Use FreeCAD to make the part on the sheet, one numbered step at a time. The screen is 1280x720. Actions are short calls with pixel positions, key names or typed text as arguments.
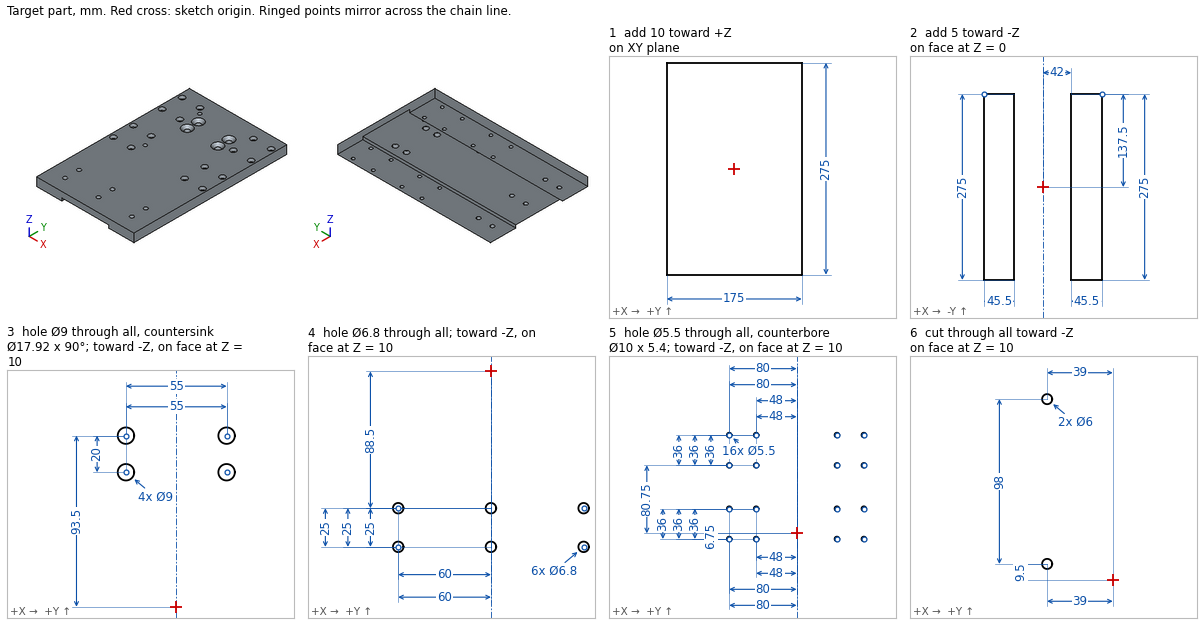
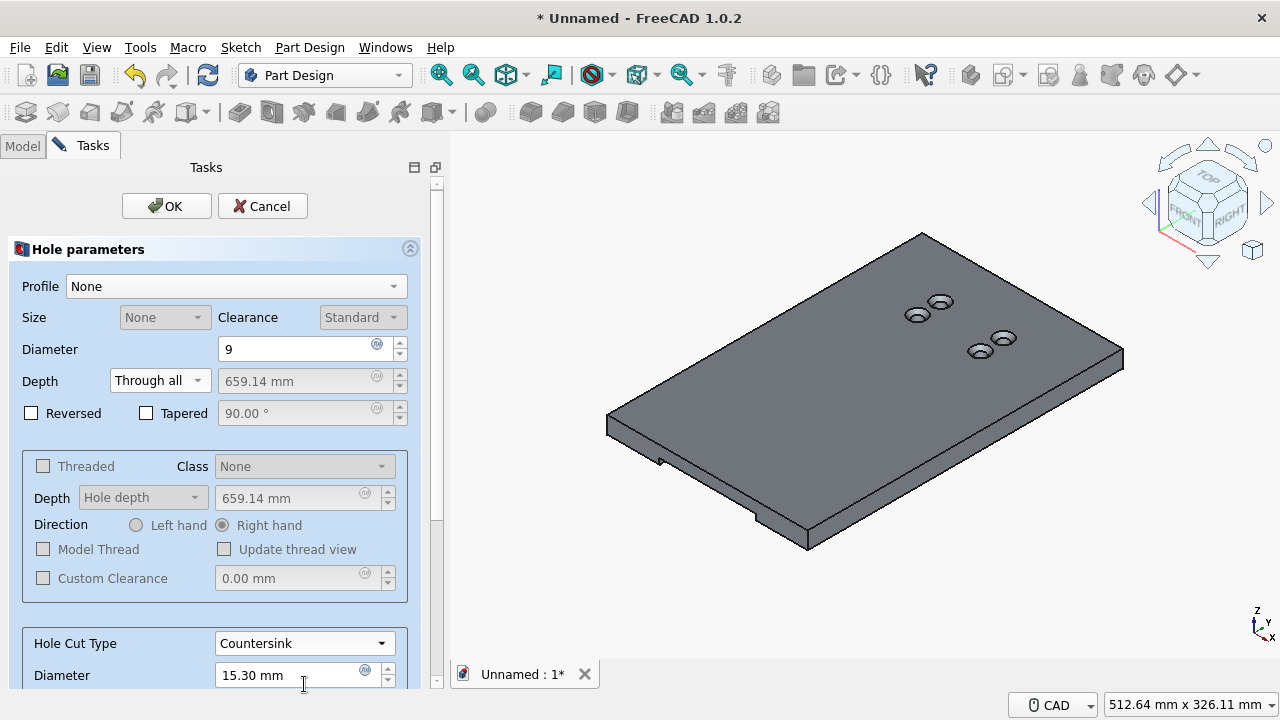
triple_click(298, 675)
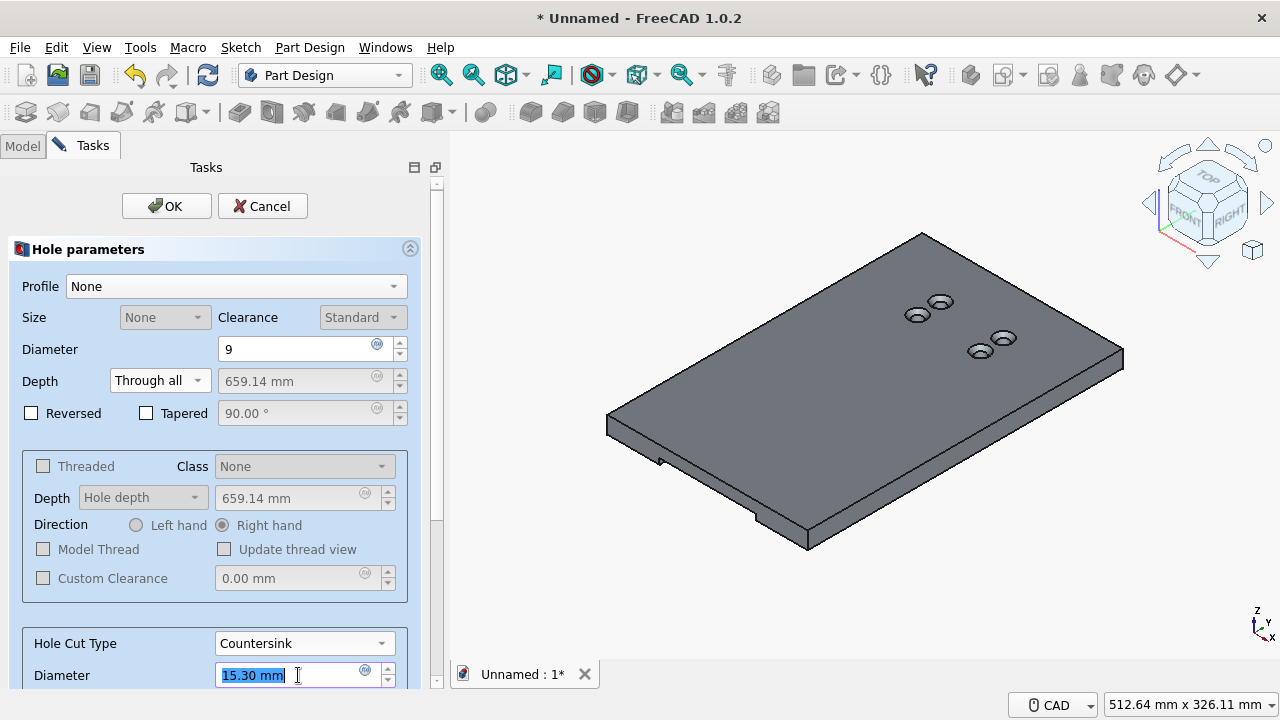
text(17.92)
key(Tab)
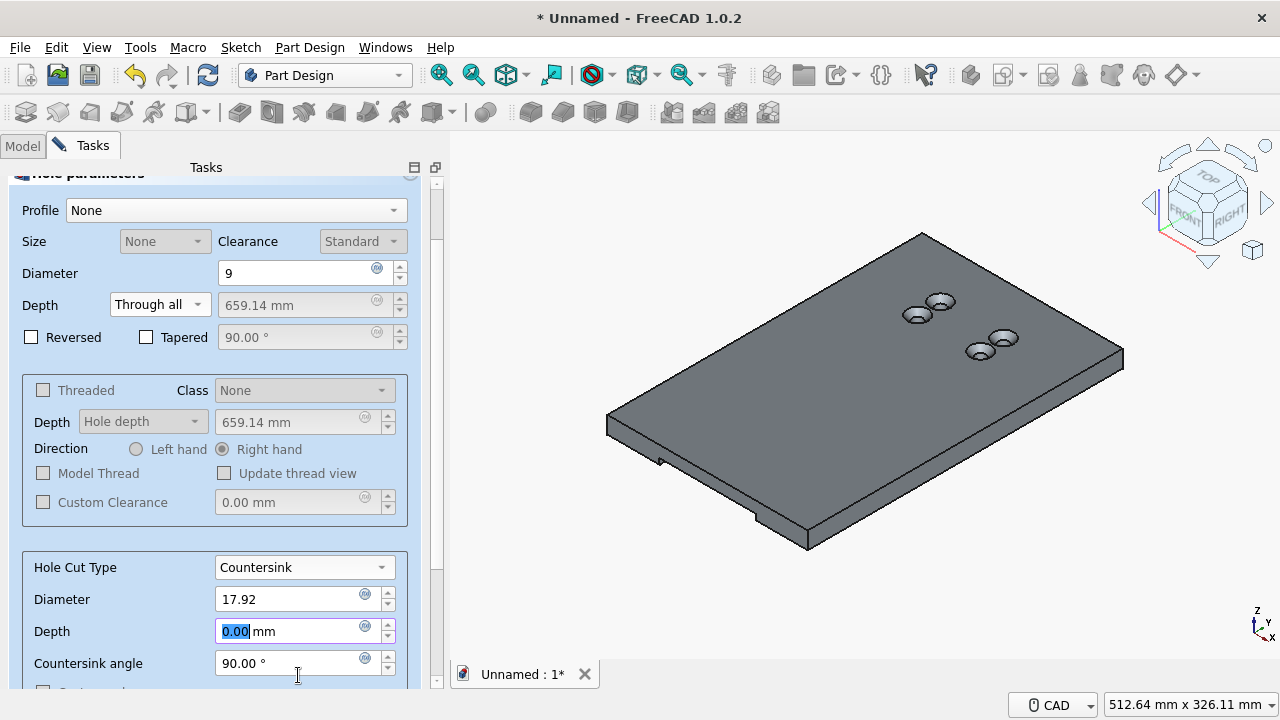
scroll(437, 432, up, 3)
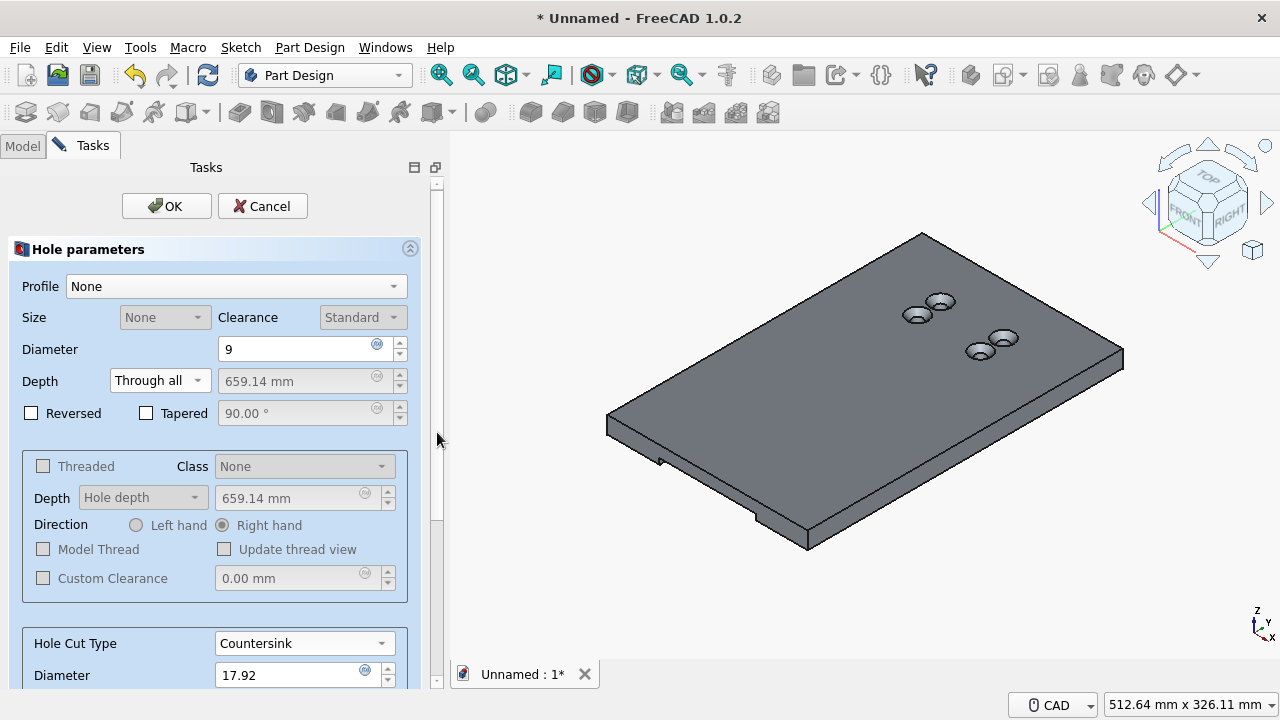
click(167, 206)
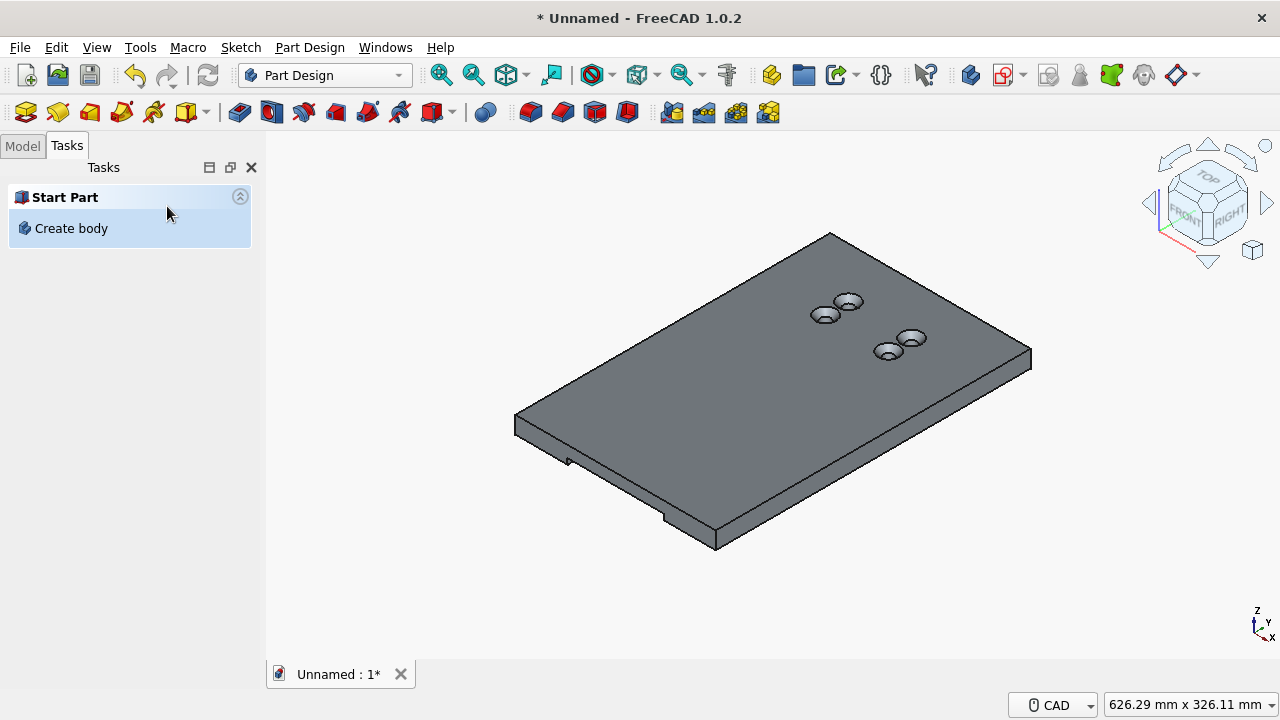
click(728, 407)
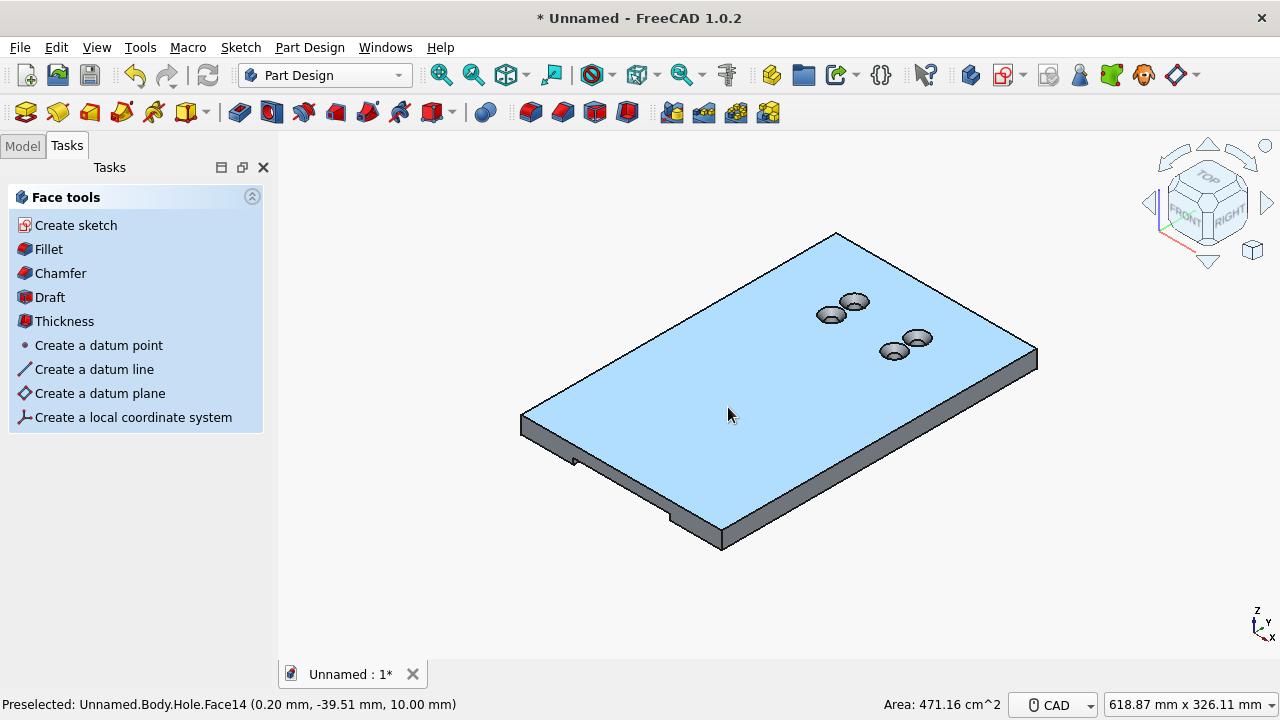
click(1004, 76)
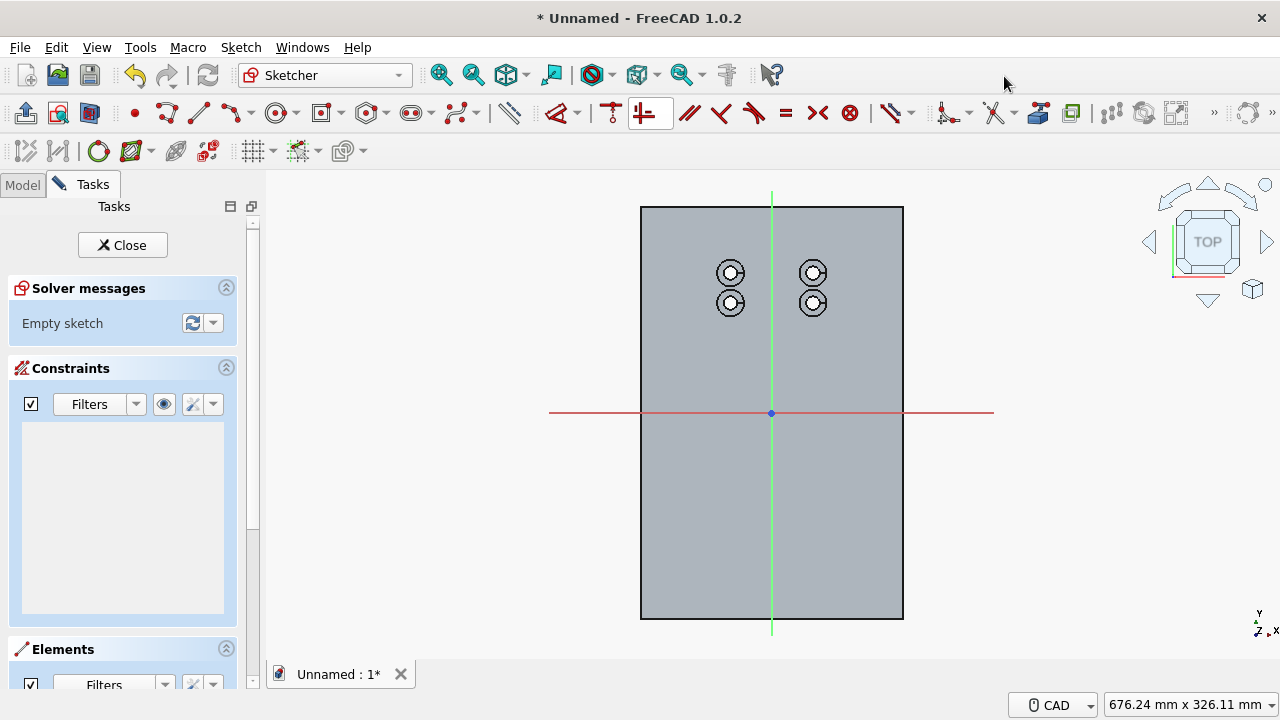
scroll(854, 606, up, 3)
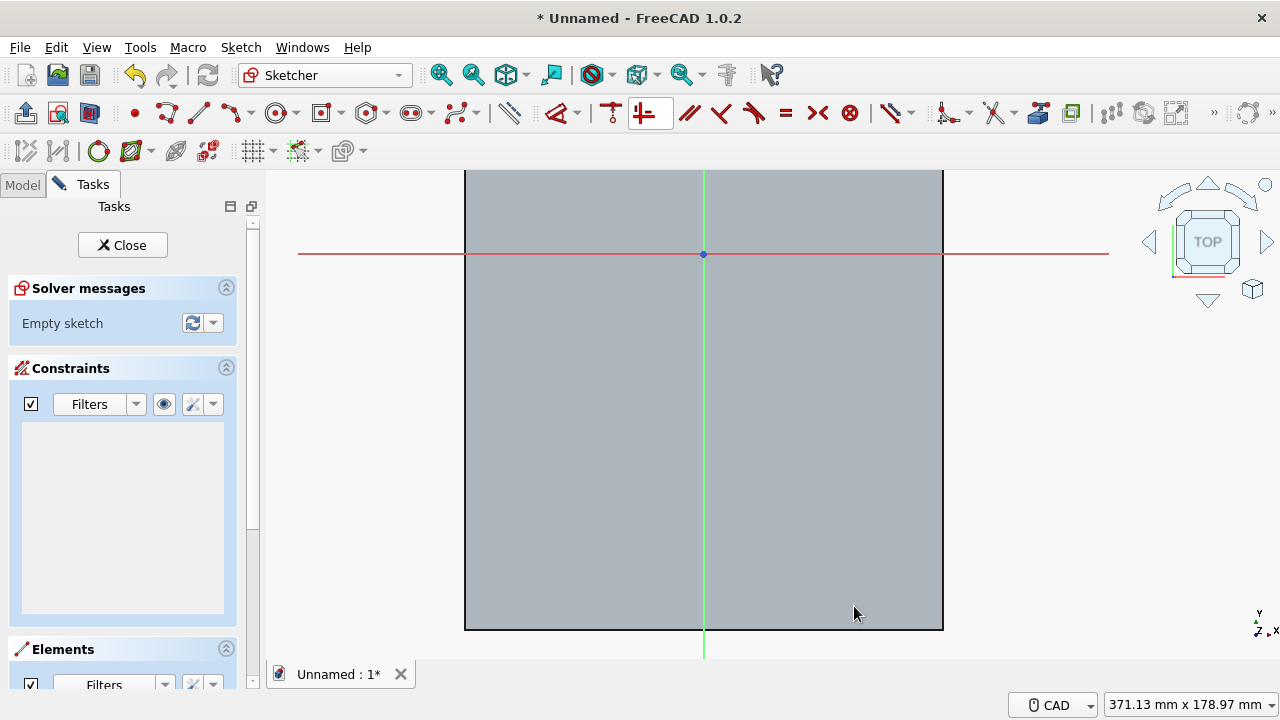
key(g)
key(c)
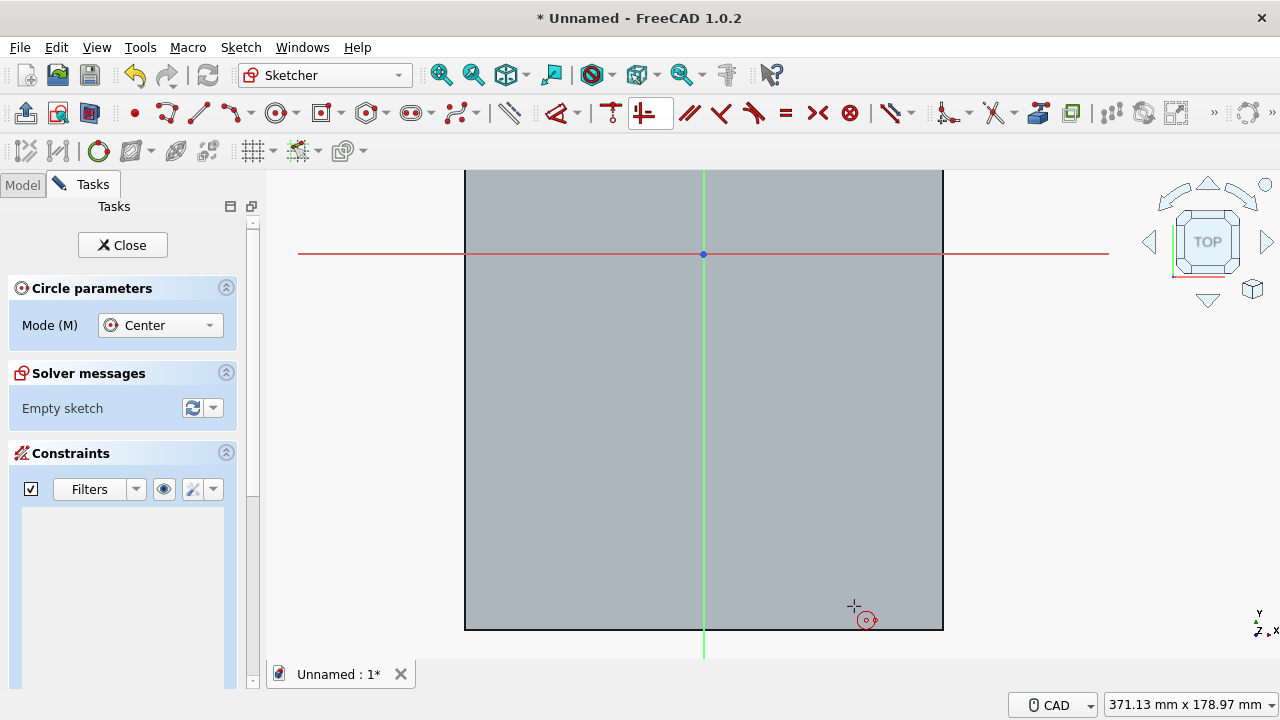
scroll(704, 564, up, 5)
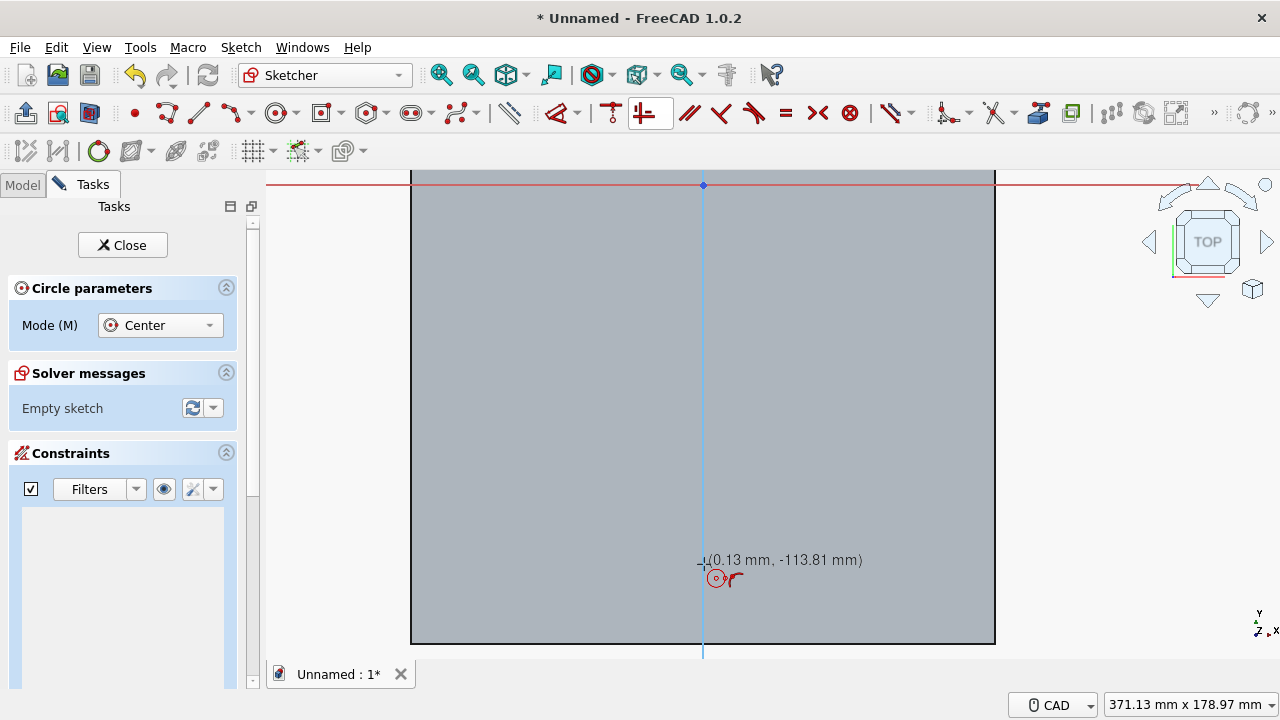
click(702, 563)
move(720, 545)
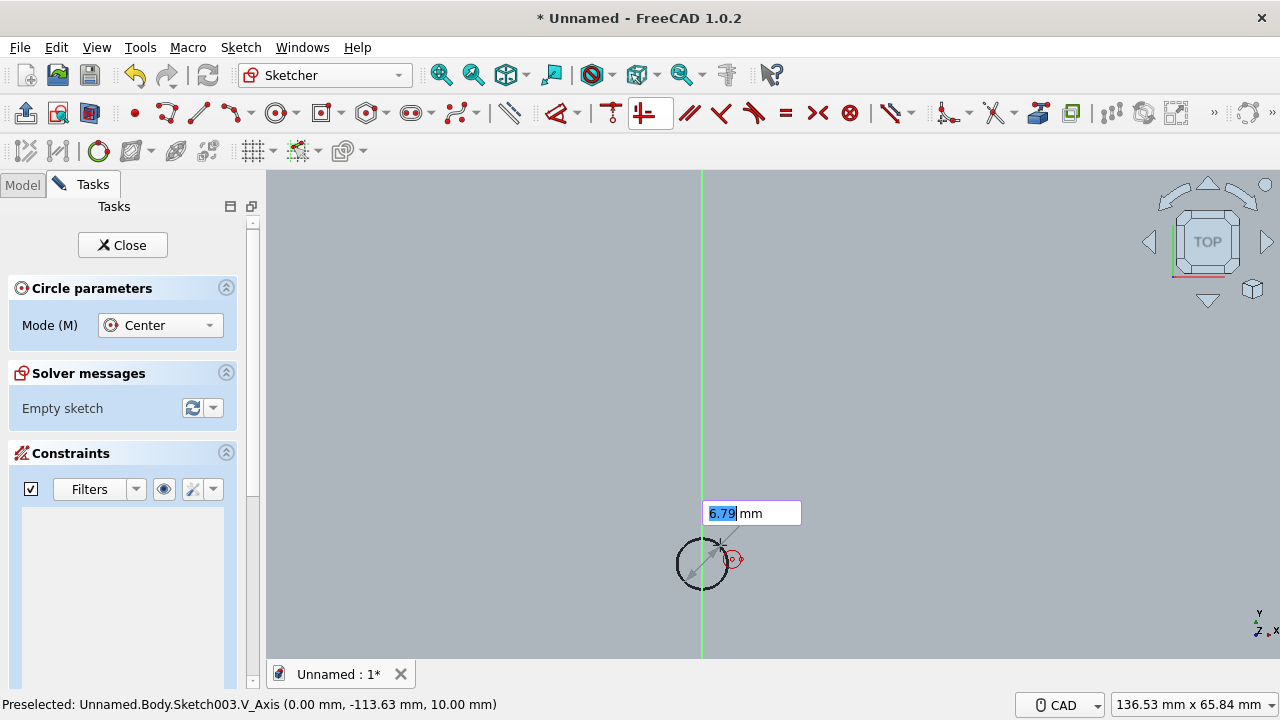
text(6.8)
key(Return)